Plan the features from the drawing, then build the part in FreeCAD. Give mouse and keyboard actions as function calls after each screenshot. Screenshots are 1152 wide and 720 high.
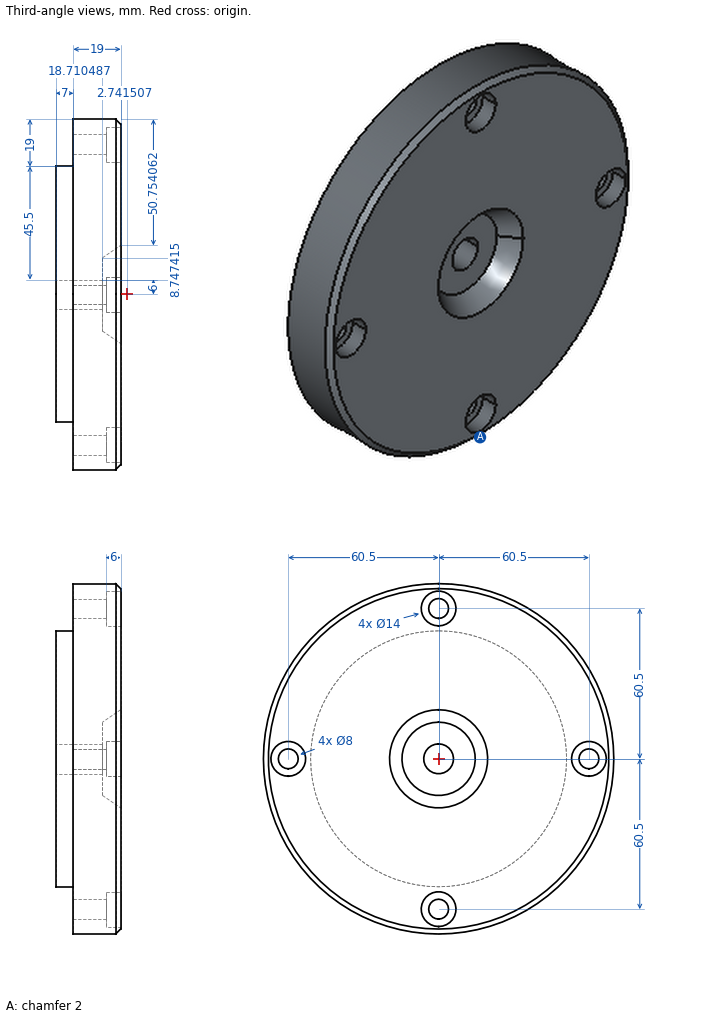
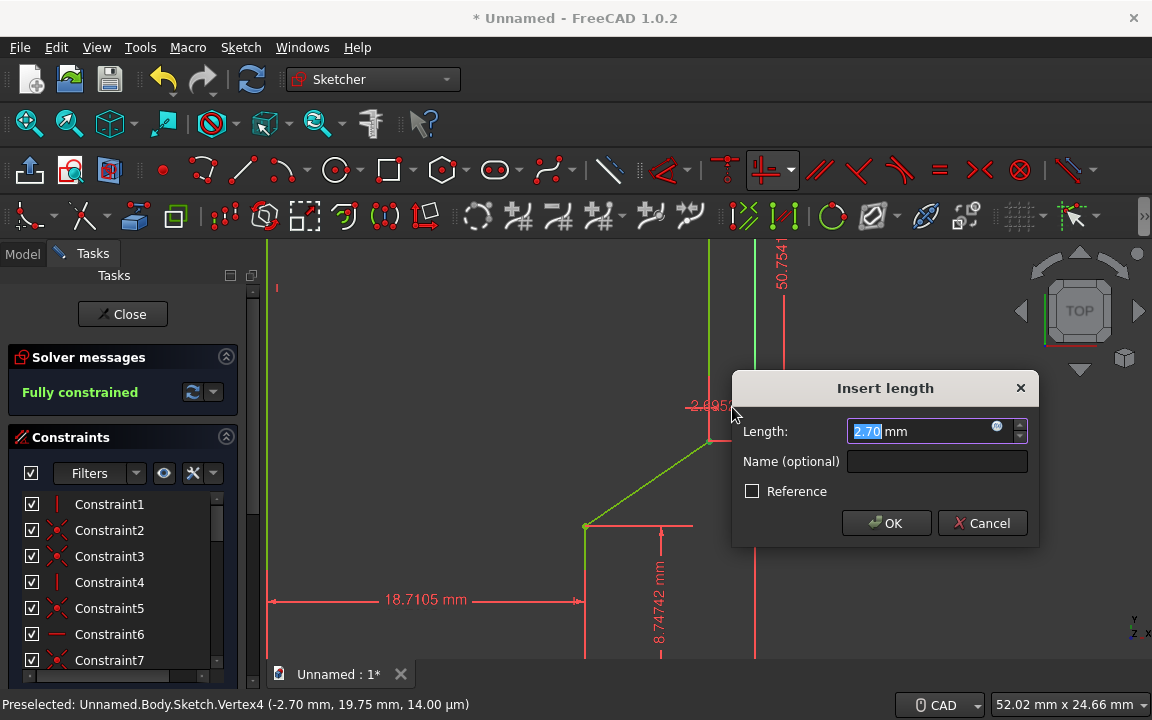
text(2.741507)
key(Return)
key(Escape)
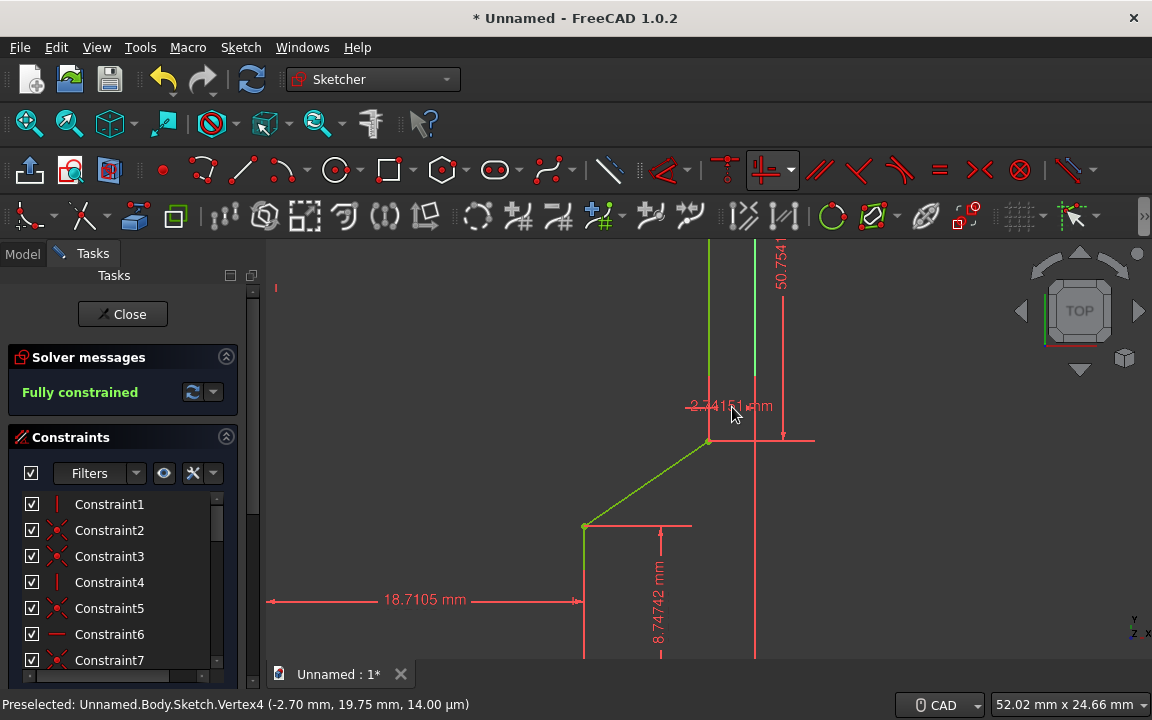
click(123, 314)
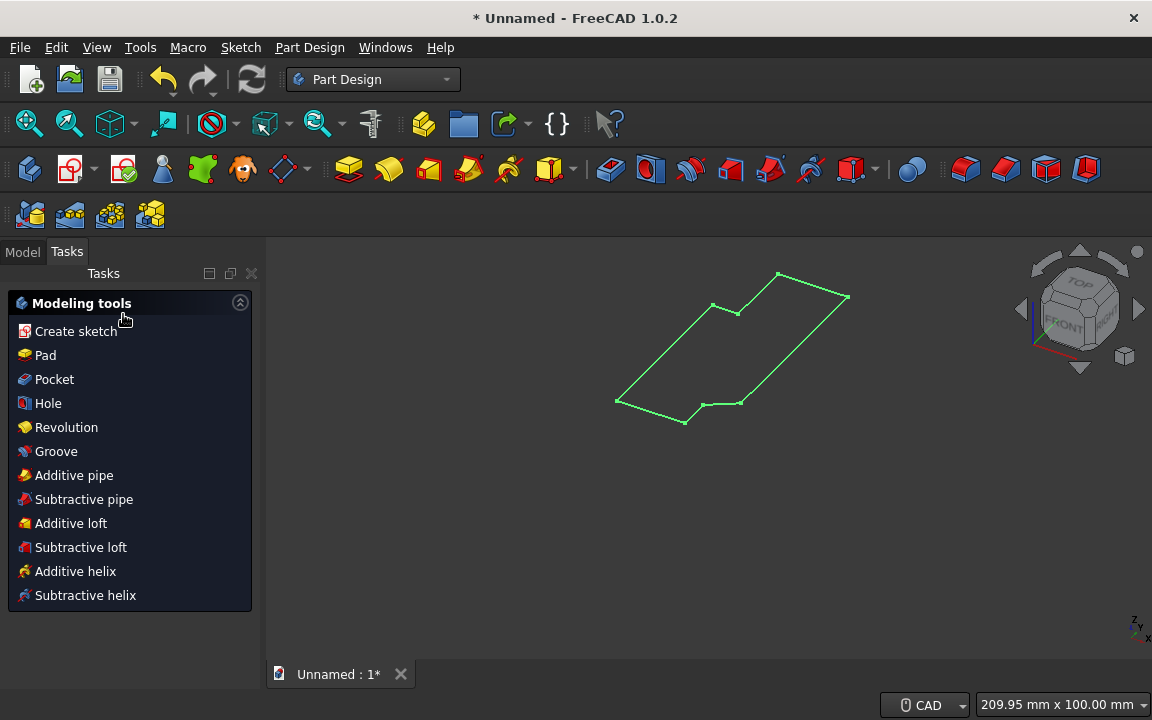
click(390, 170)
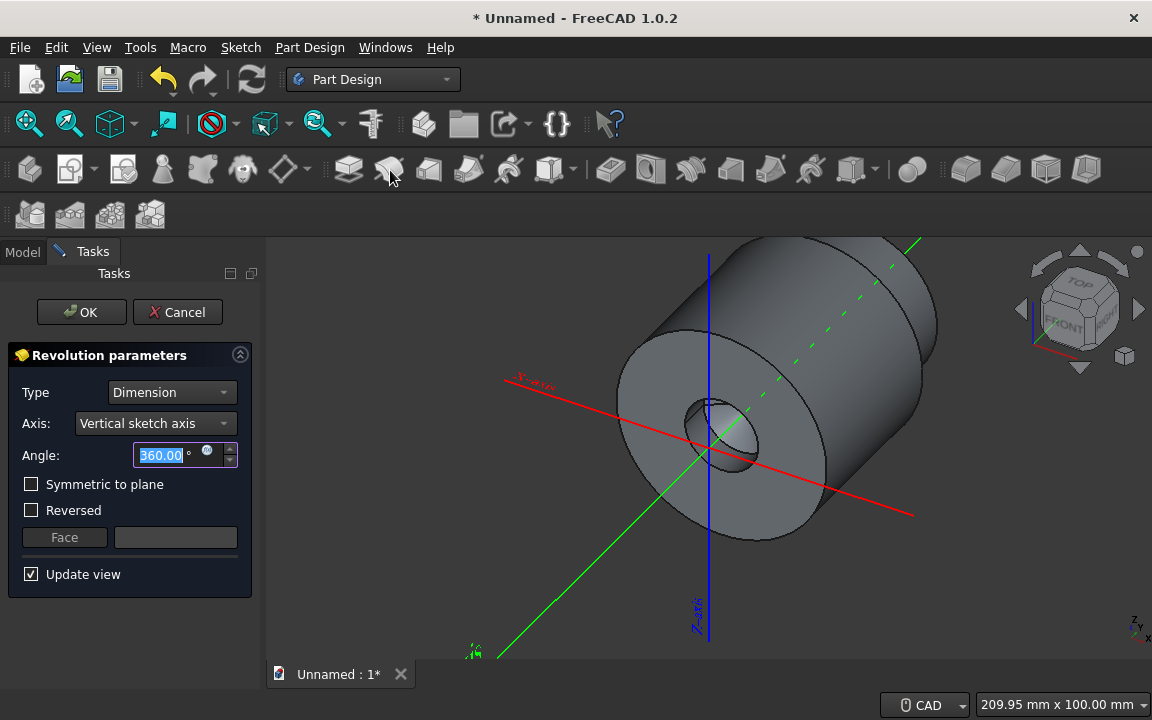
click(156, 424)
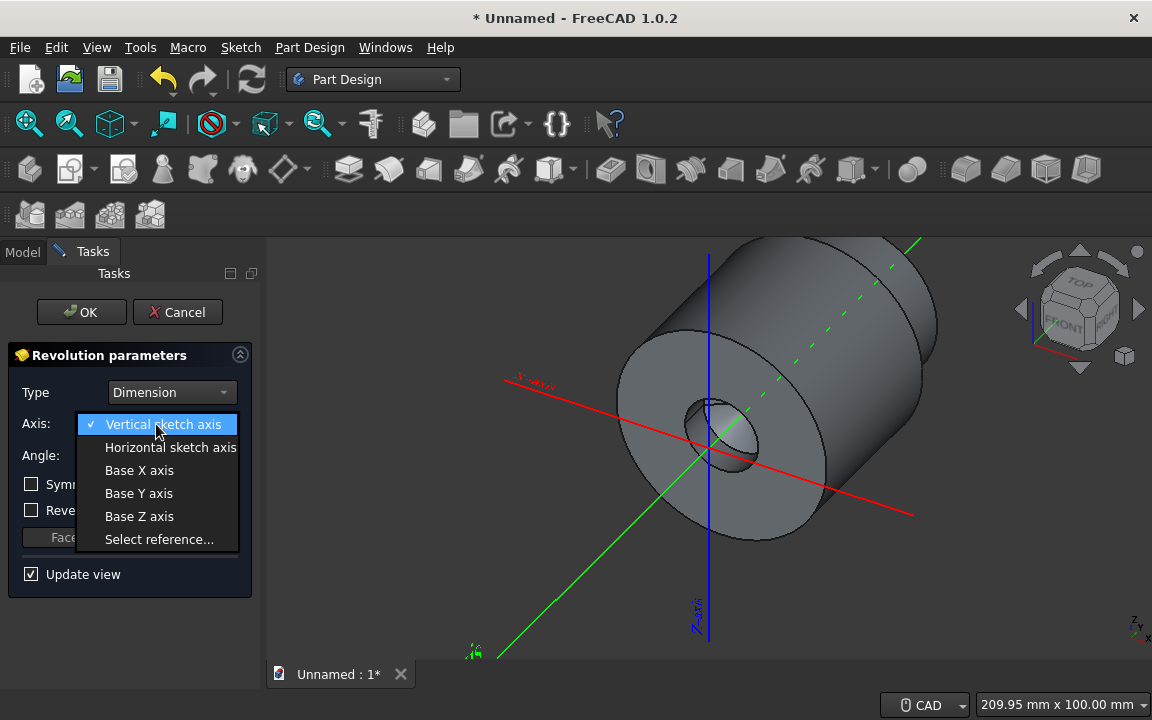
click(156, 448)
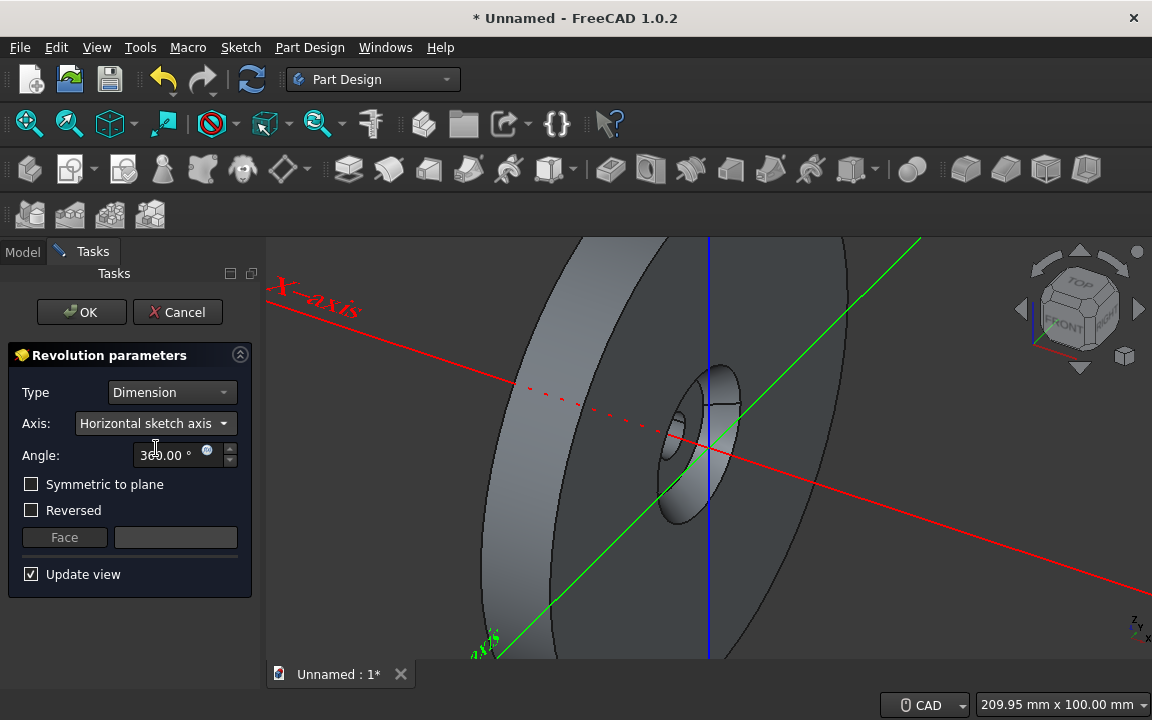
click(82, 312)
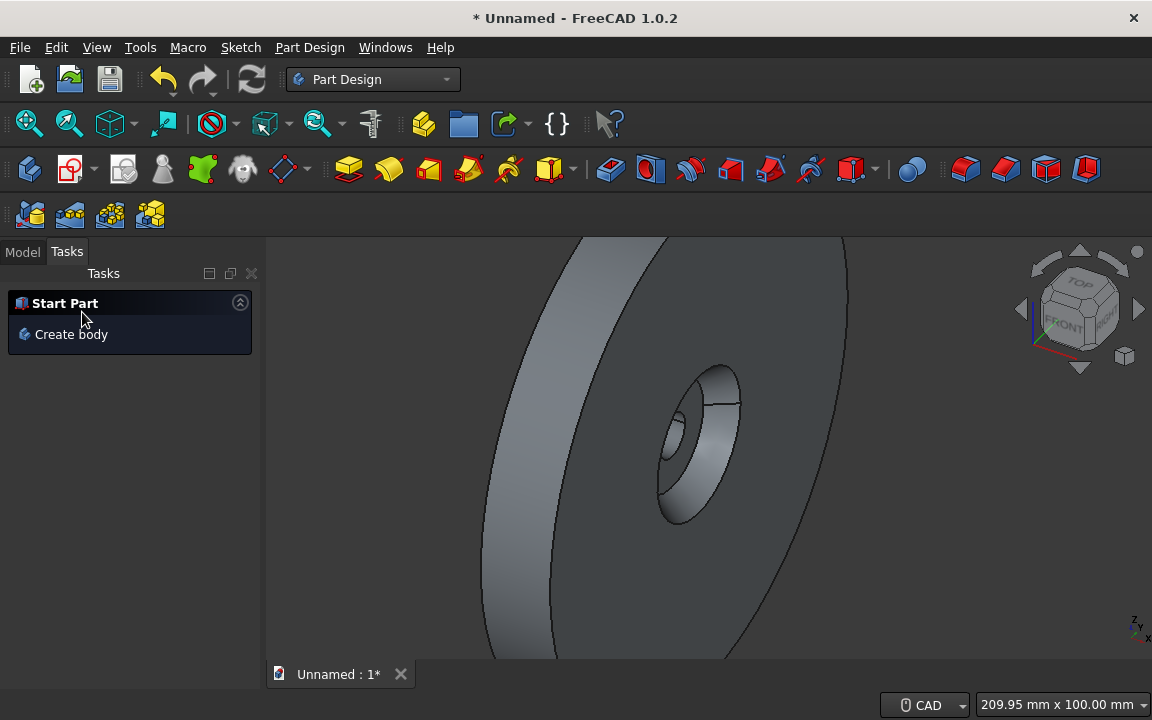
key(v)
key(f)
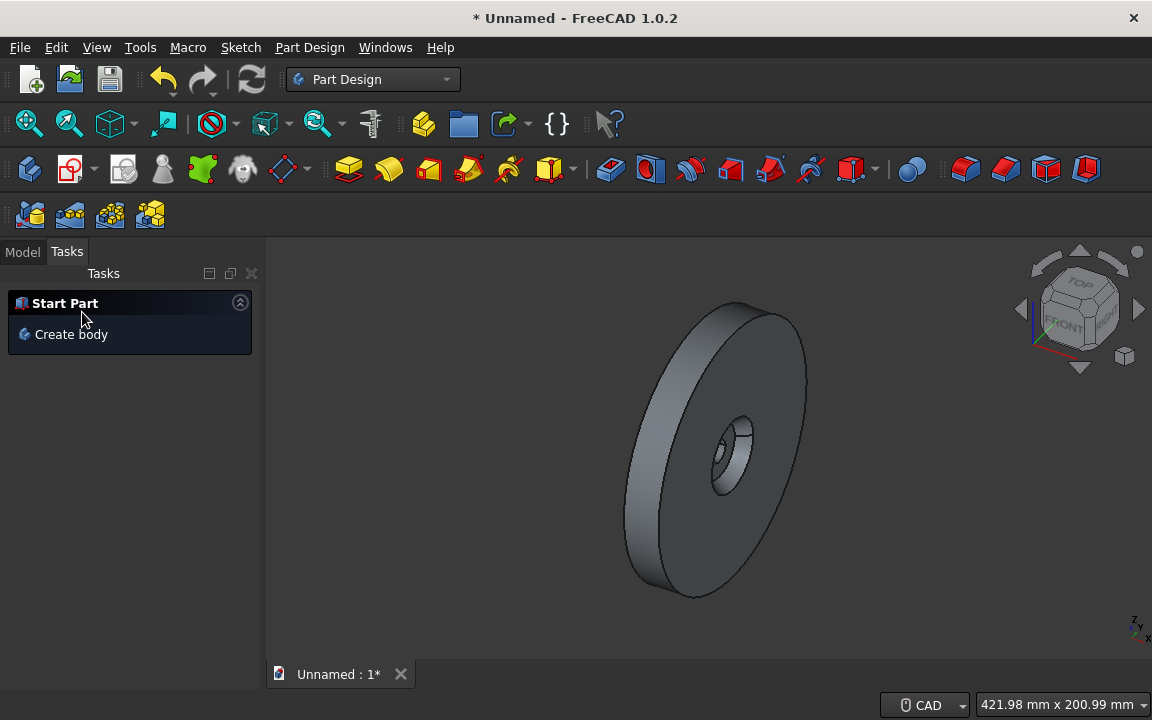
click(659, 528)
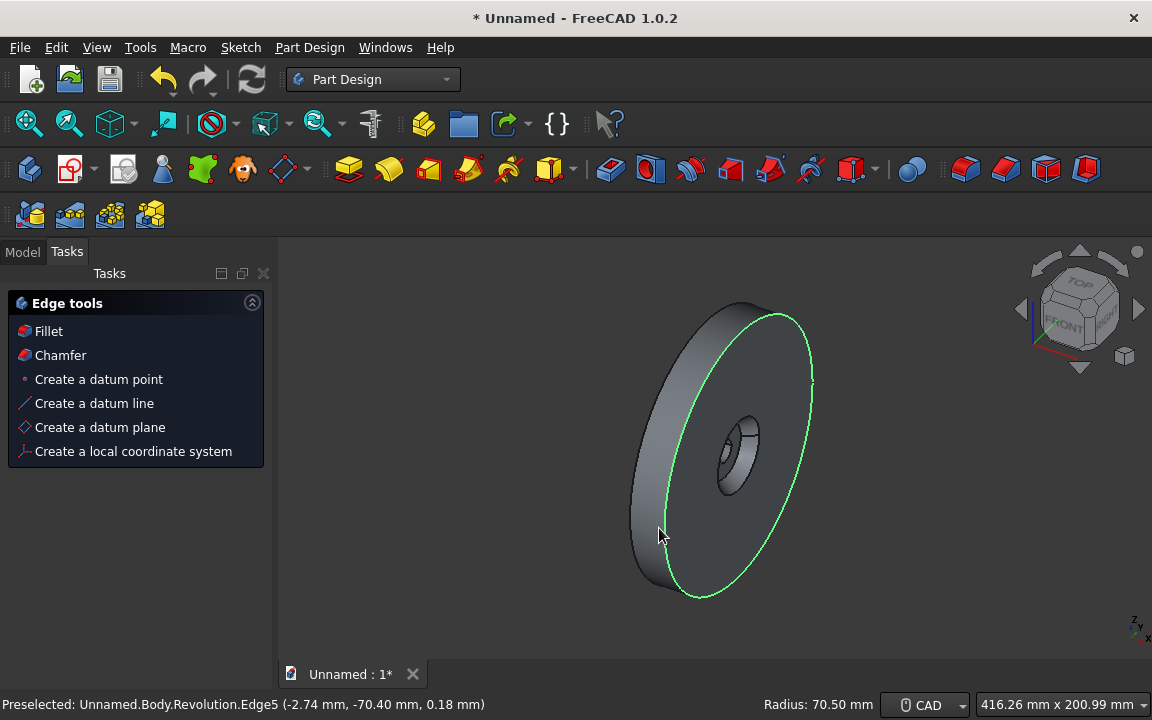
click(1006, 170)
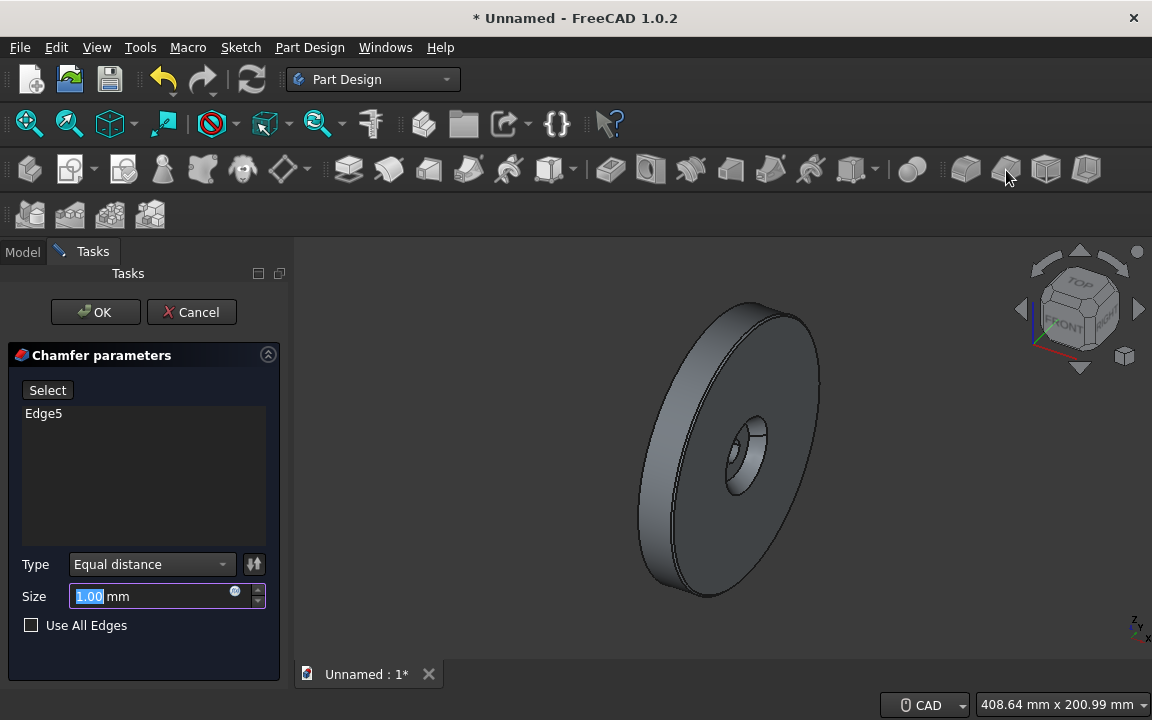
text(2)
key(Tab)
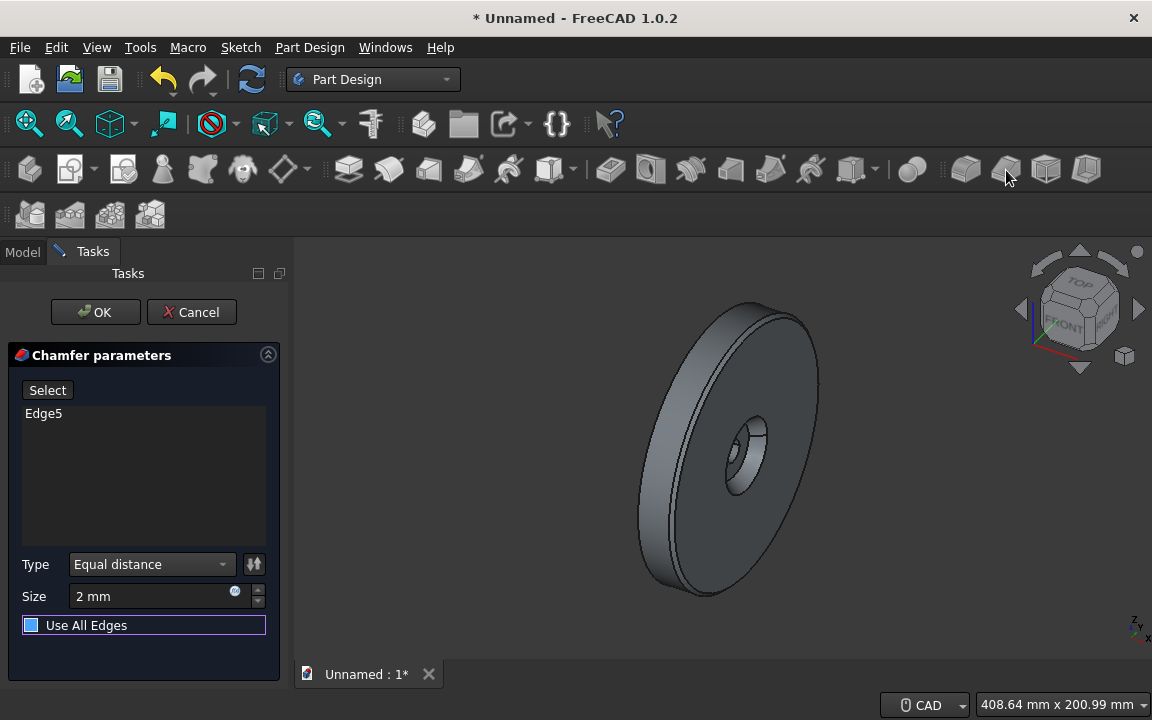
click(96, 312)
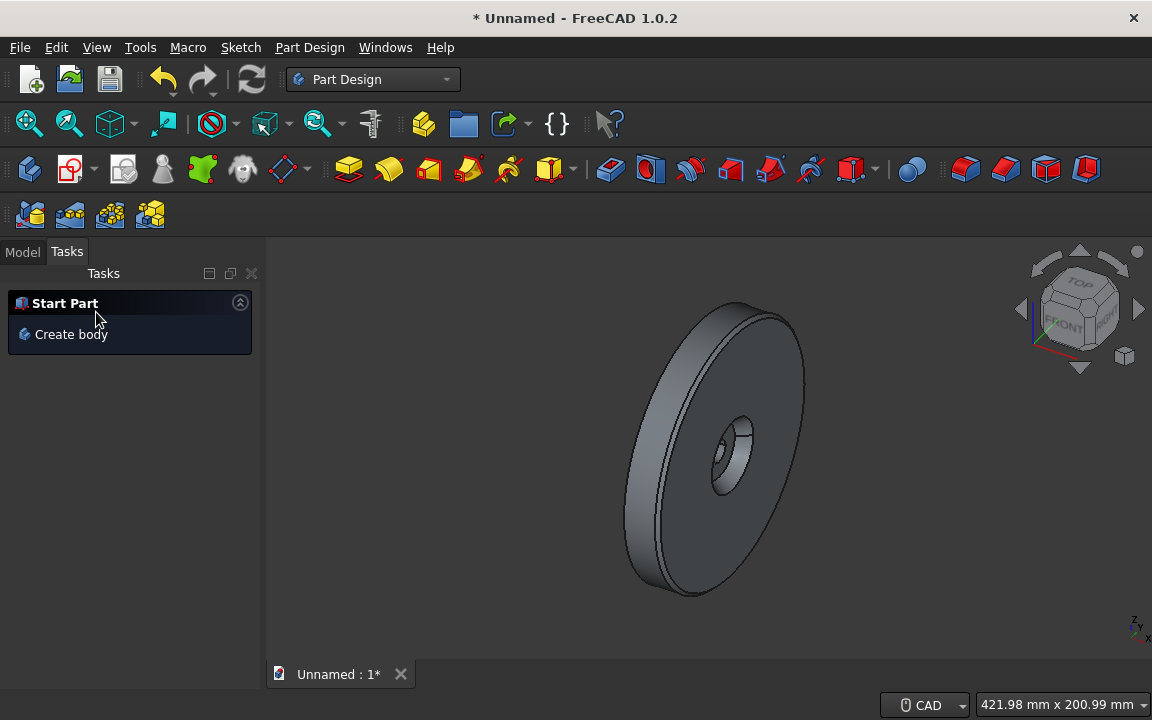
click(774, 380)